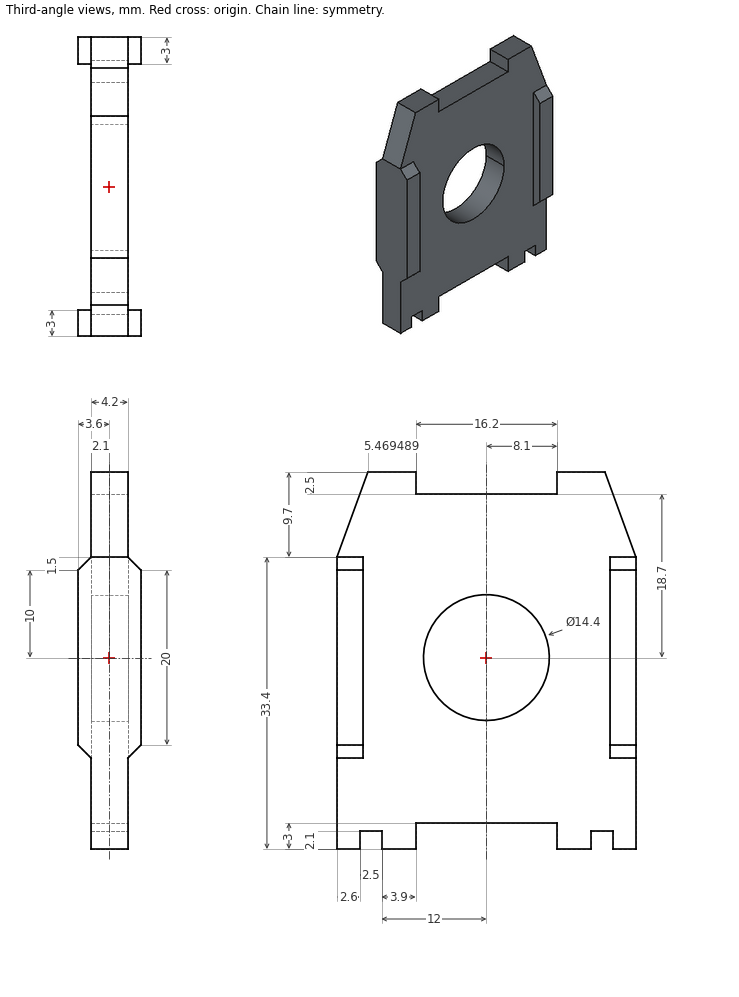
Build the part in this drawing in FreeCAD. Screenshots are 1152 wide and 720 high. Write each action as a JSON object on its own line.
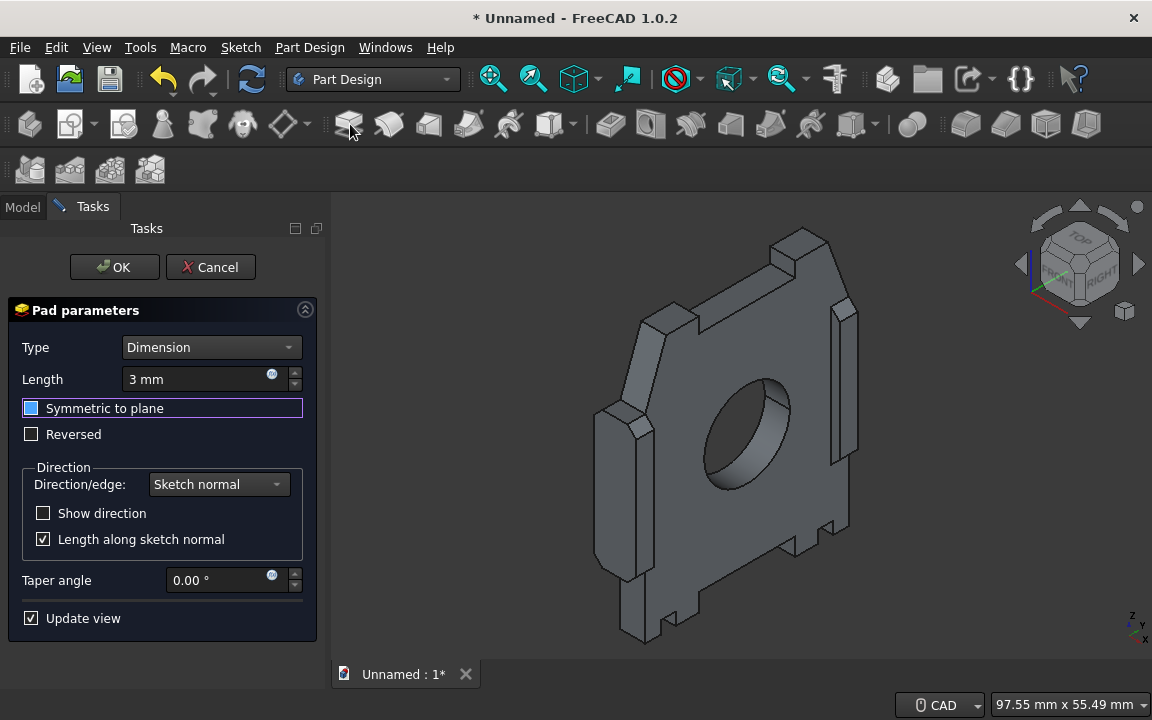
{"action": "left_click", "coordinate": [30, 434]}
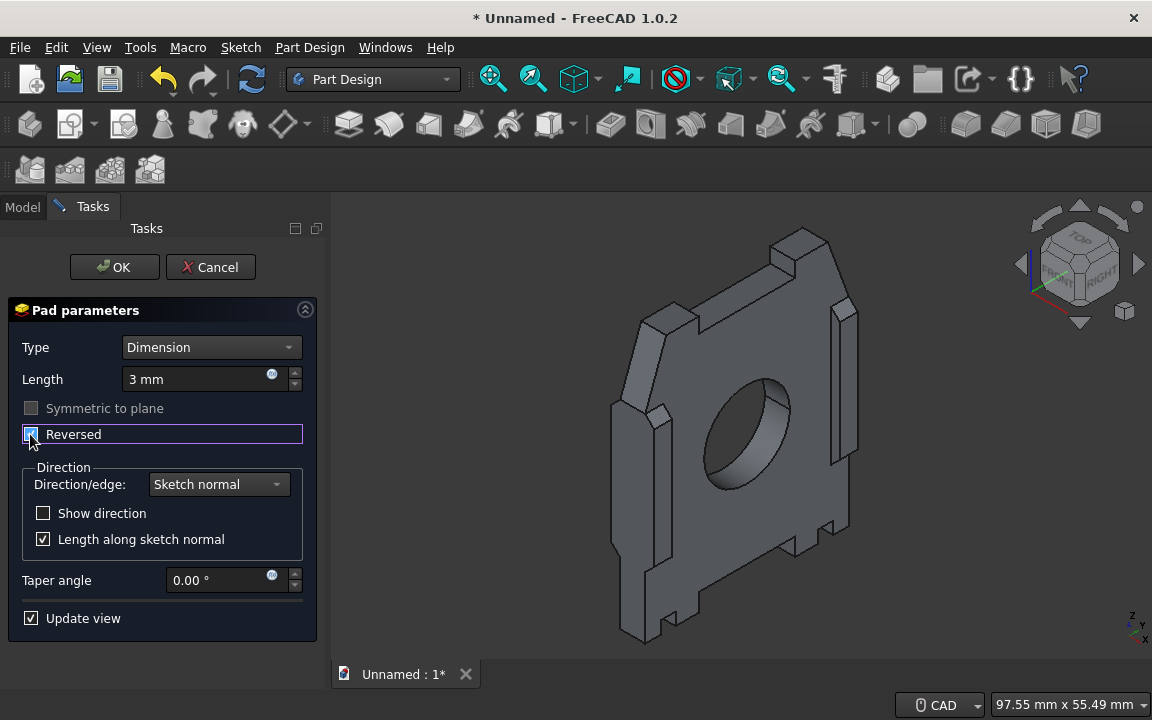
{"action": "left_click", "coordinate": [115, 267]}